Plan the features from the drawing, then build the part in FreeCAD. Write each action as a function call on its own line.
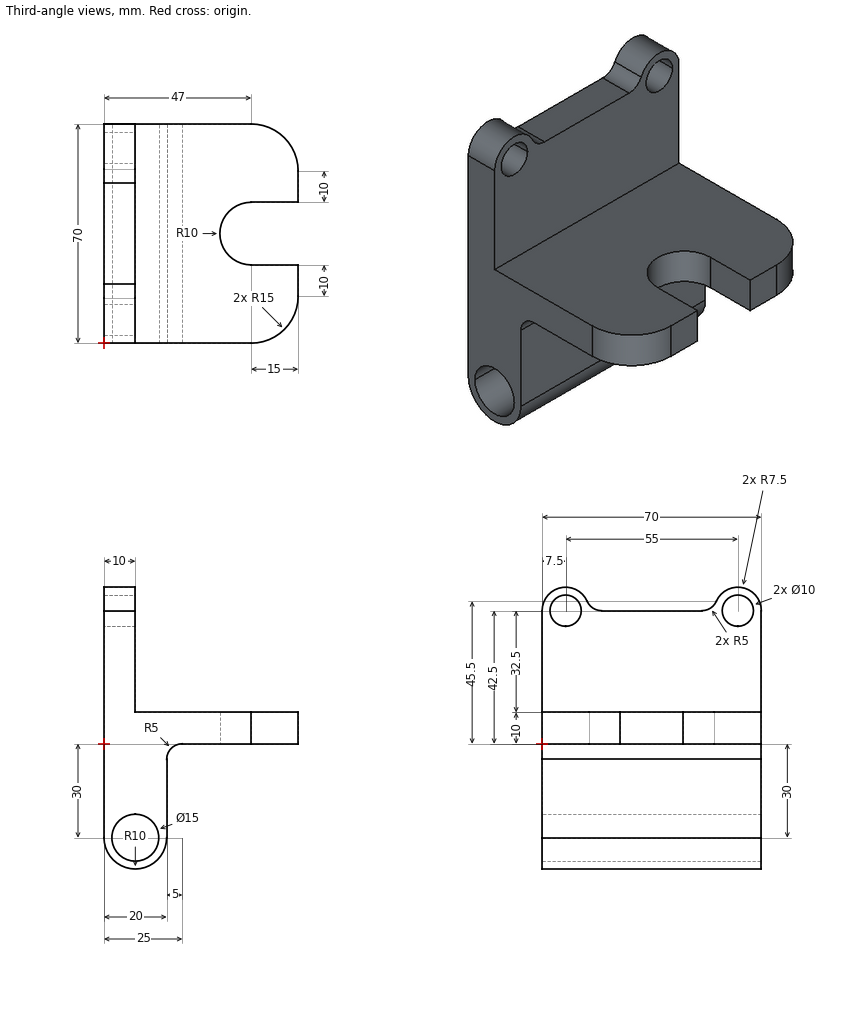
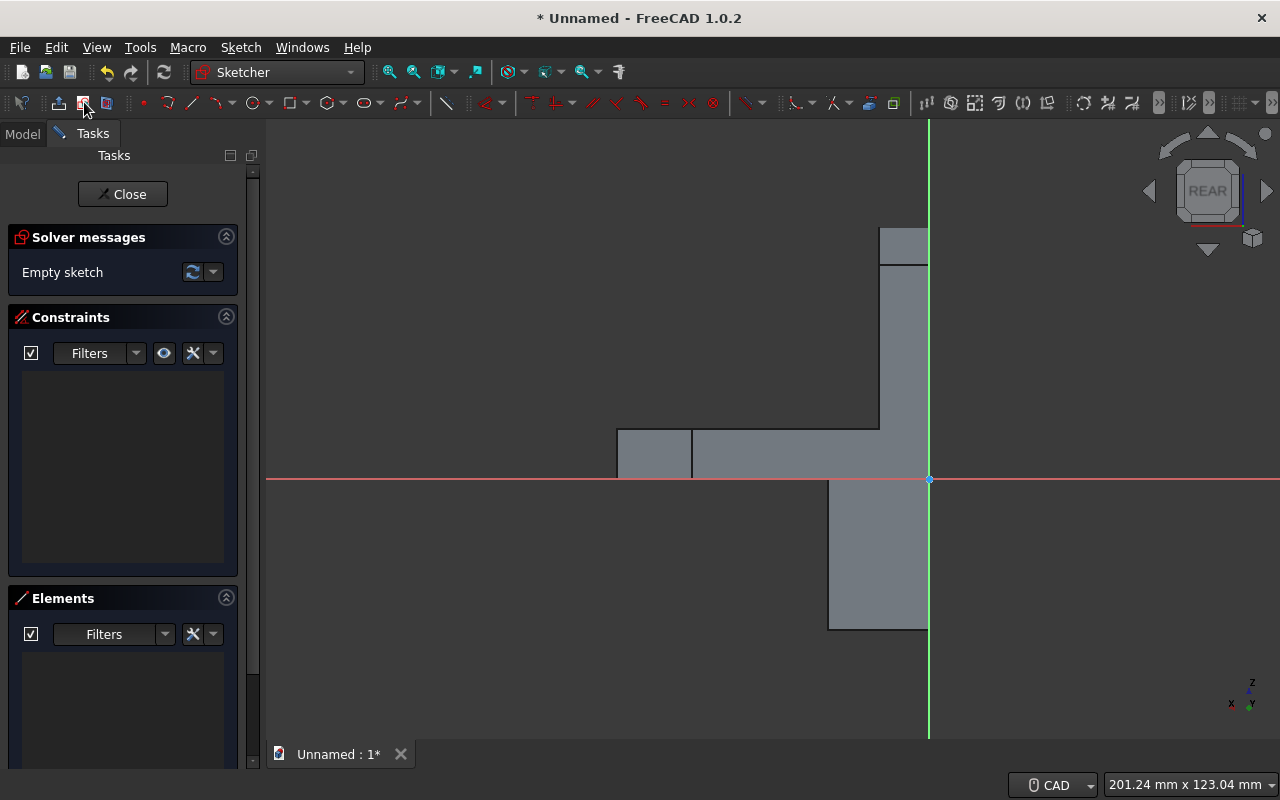
scroll(823, 496, up, 14)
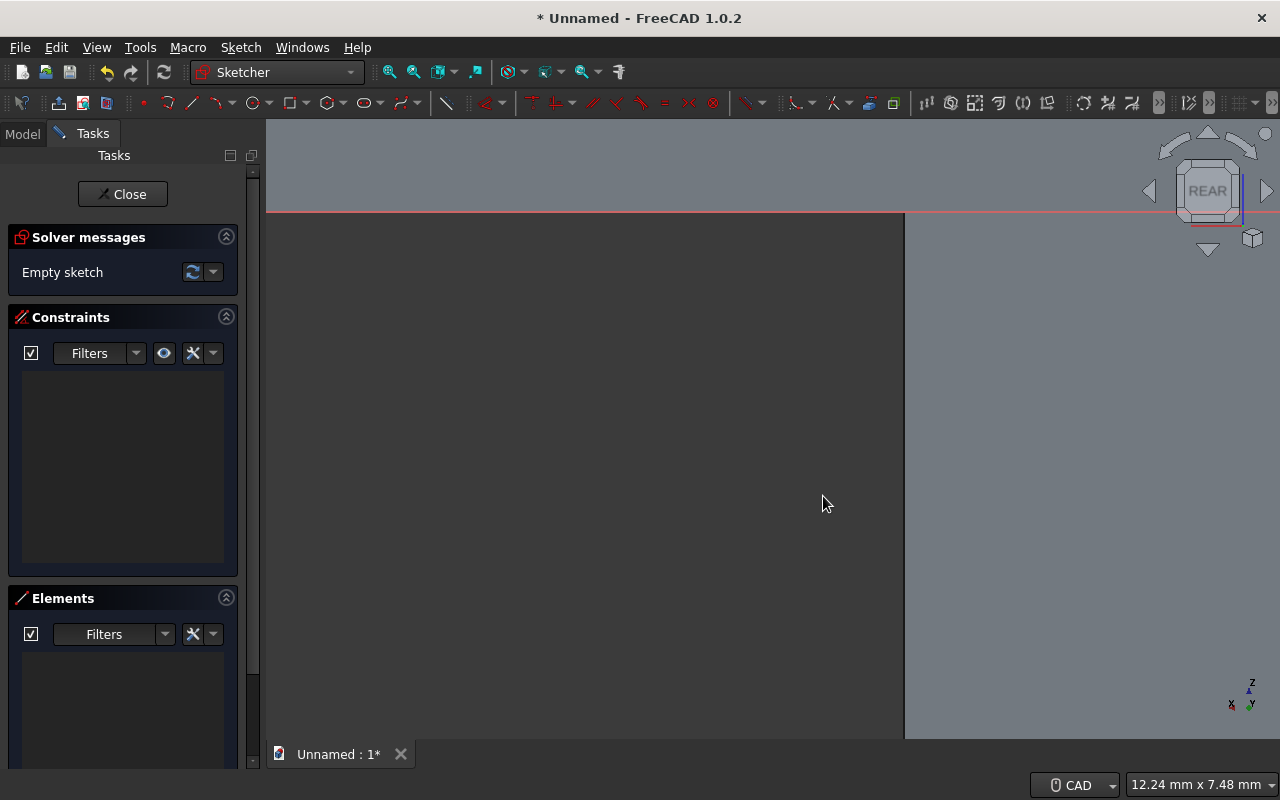
click(168, 104)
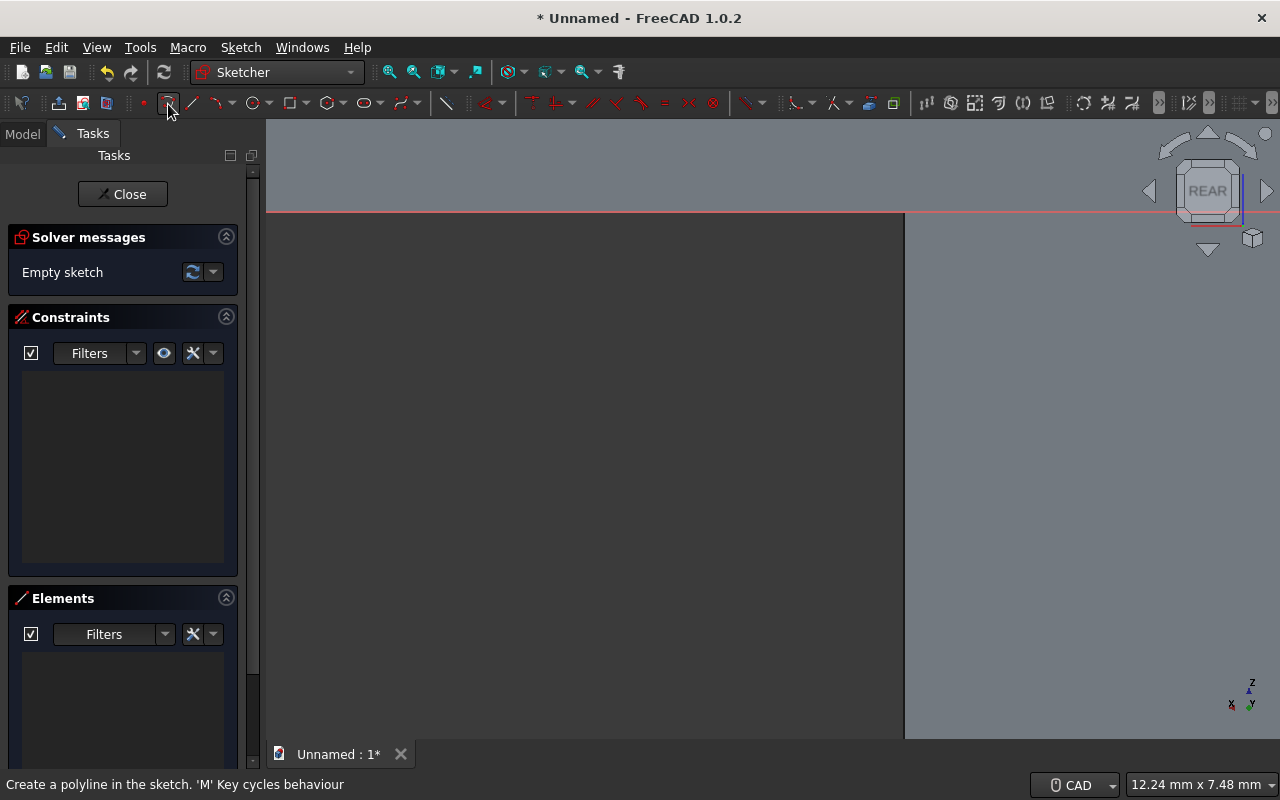
click(904, 627)
click(904, 212)
click(489, 221)
right_click(489, 221)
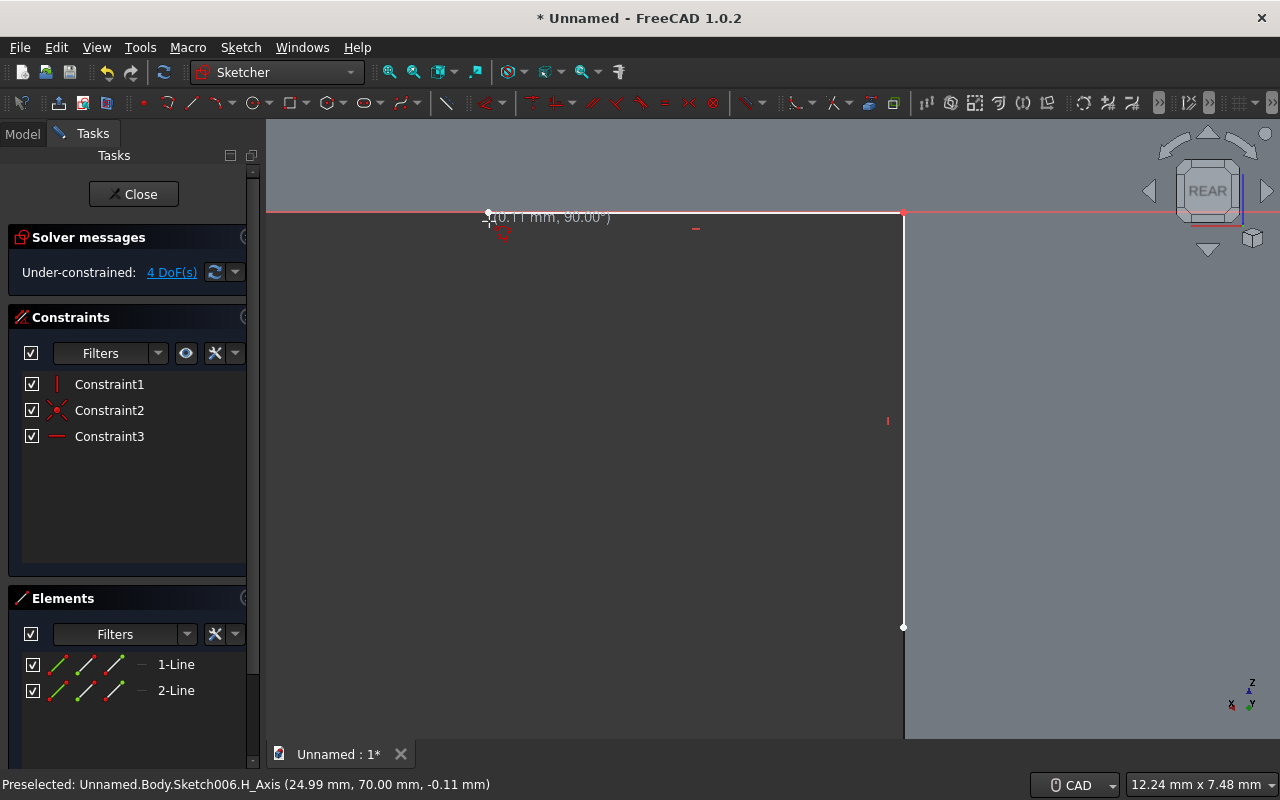
click(216, 104)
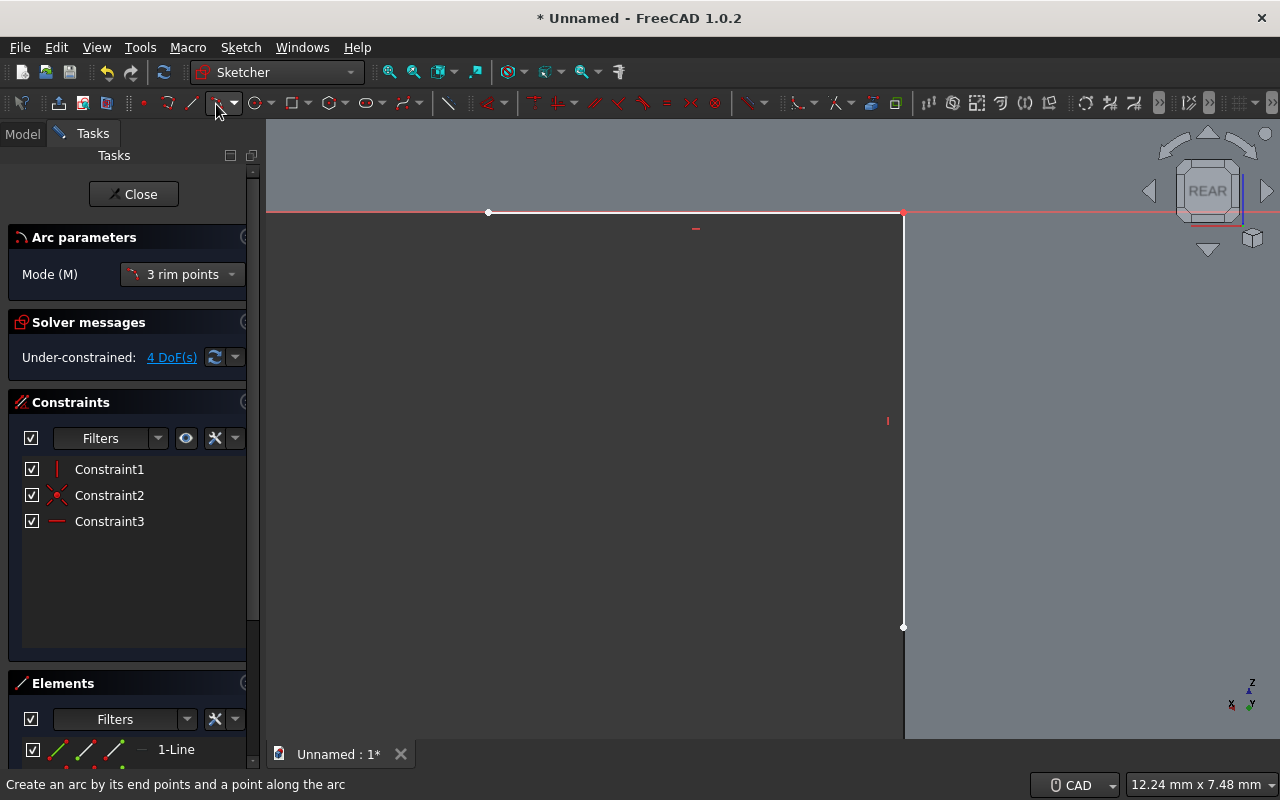
click(489, 213)
click(904, 628)
click(782, 334)
key(Escape)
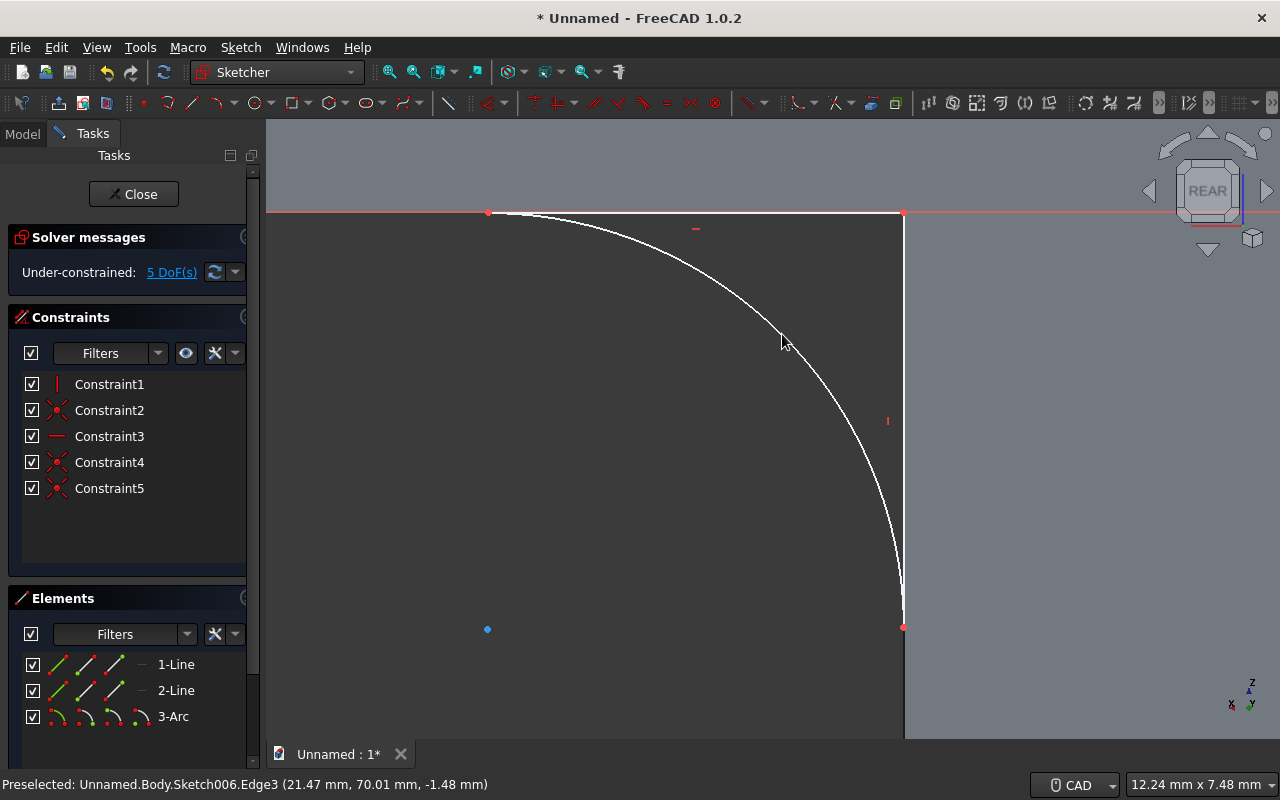
click(904, 503)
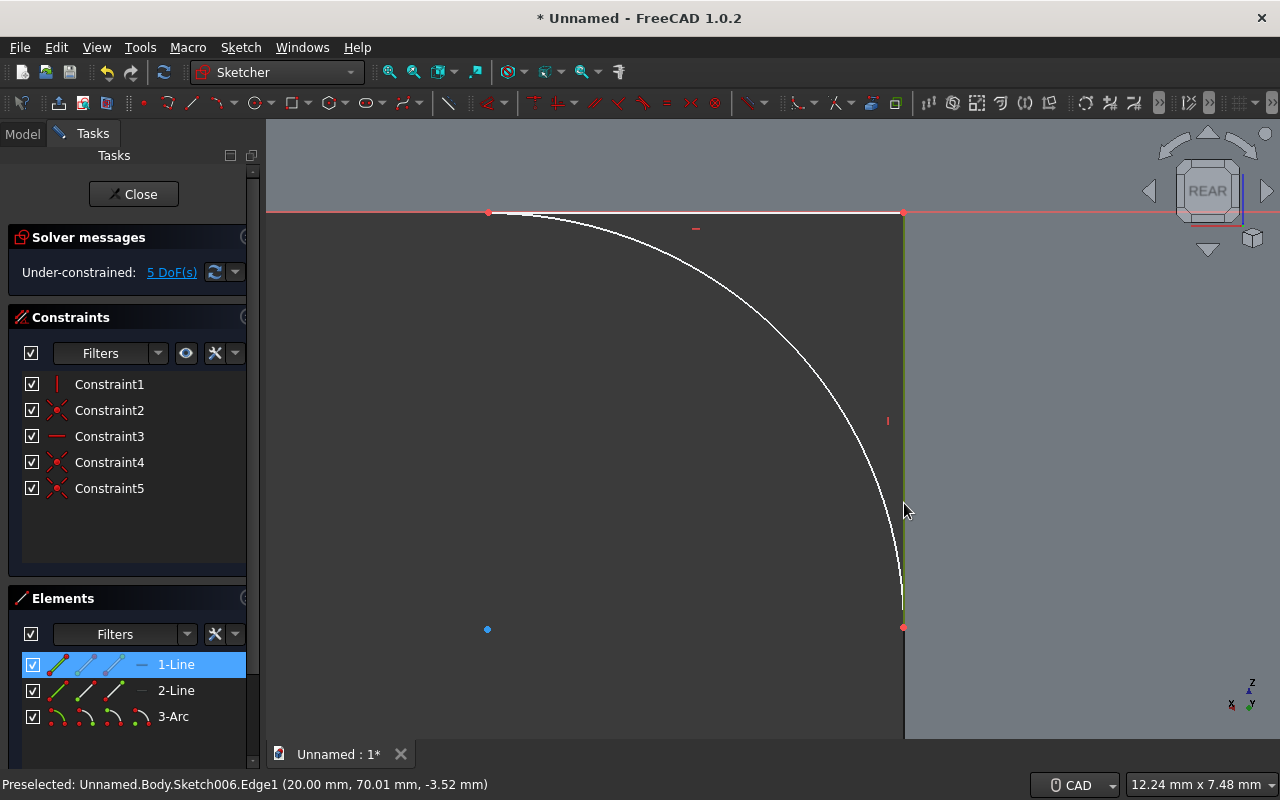
click(858, 440)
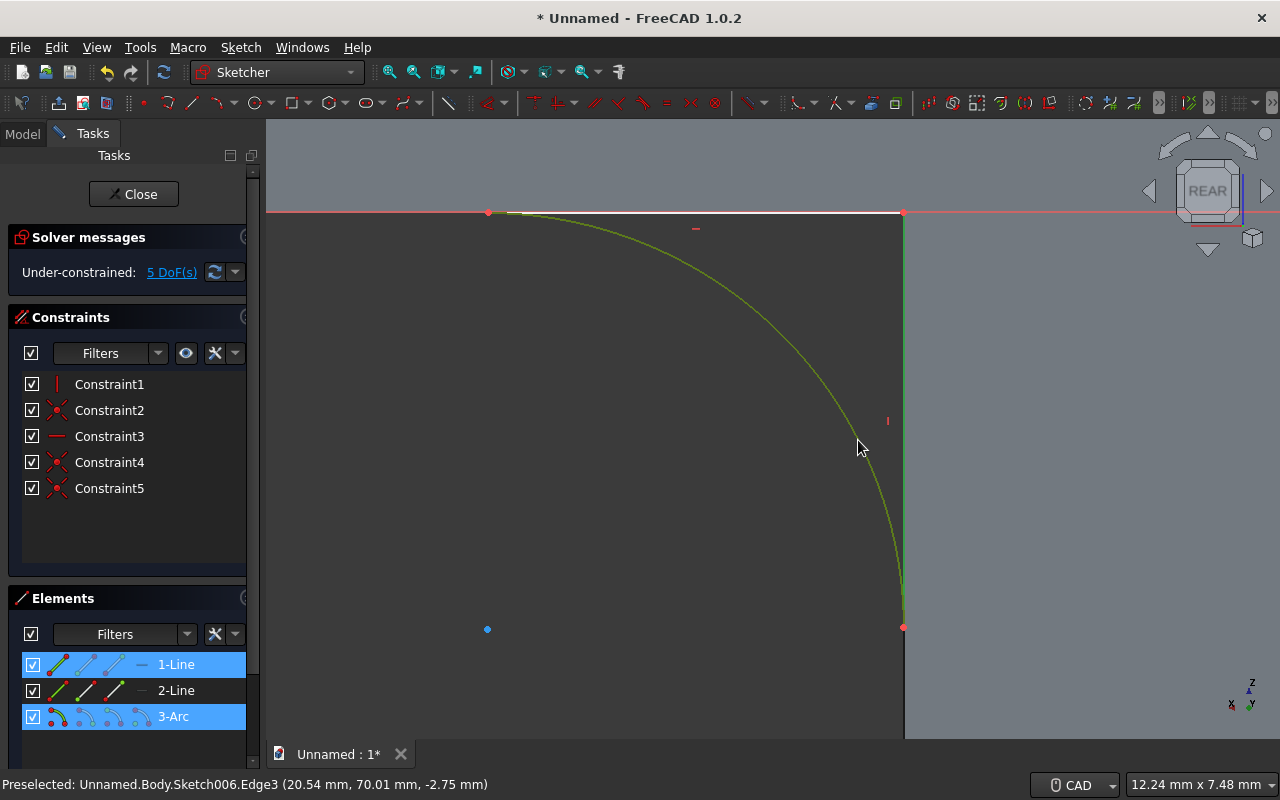
click(644, 104)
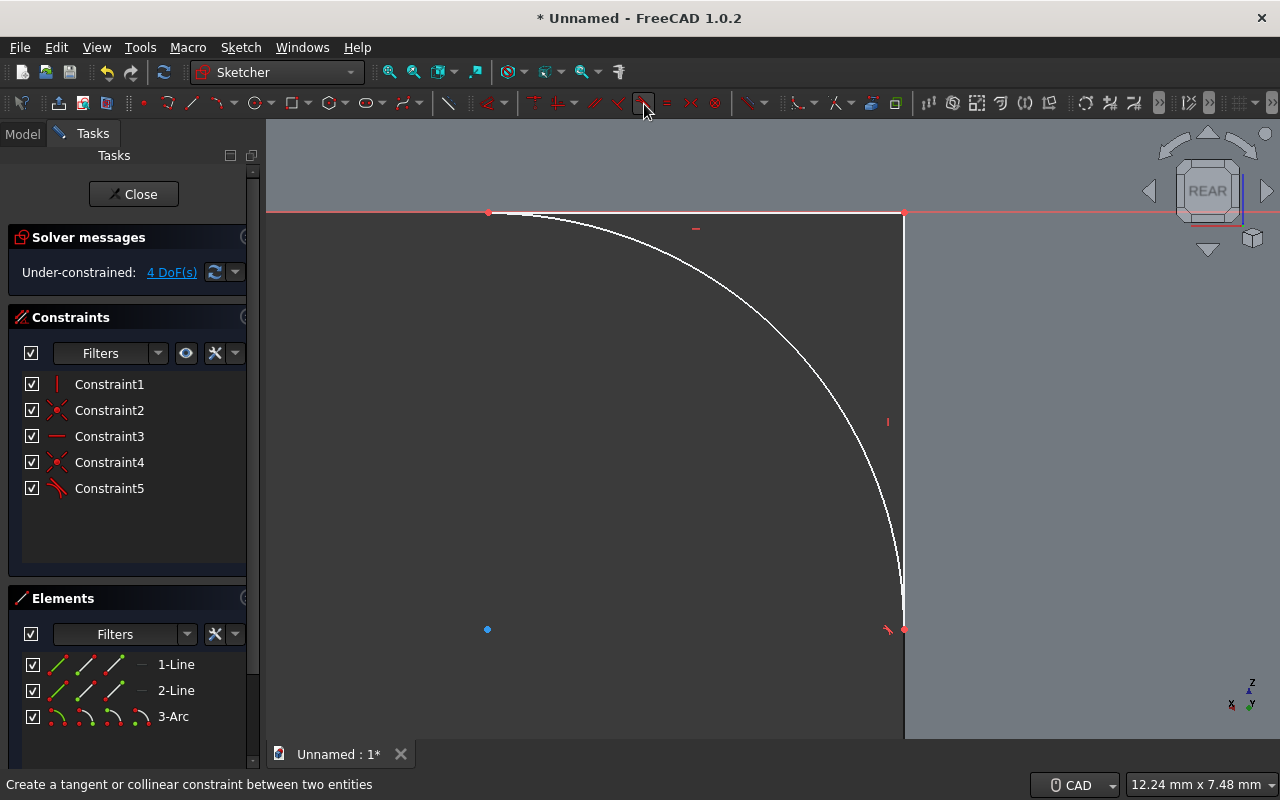
click(780, 213)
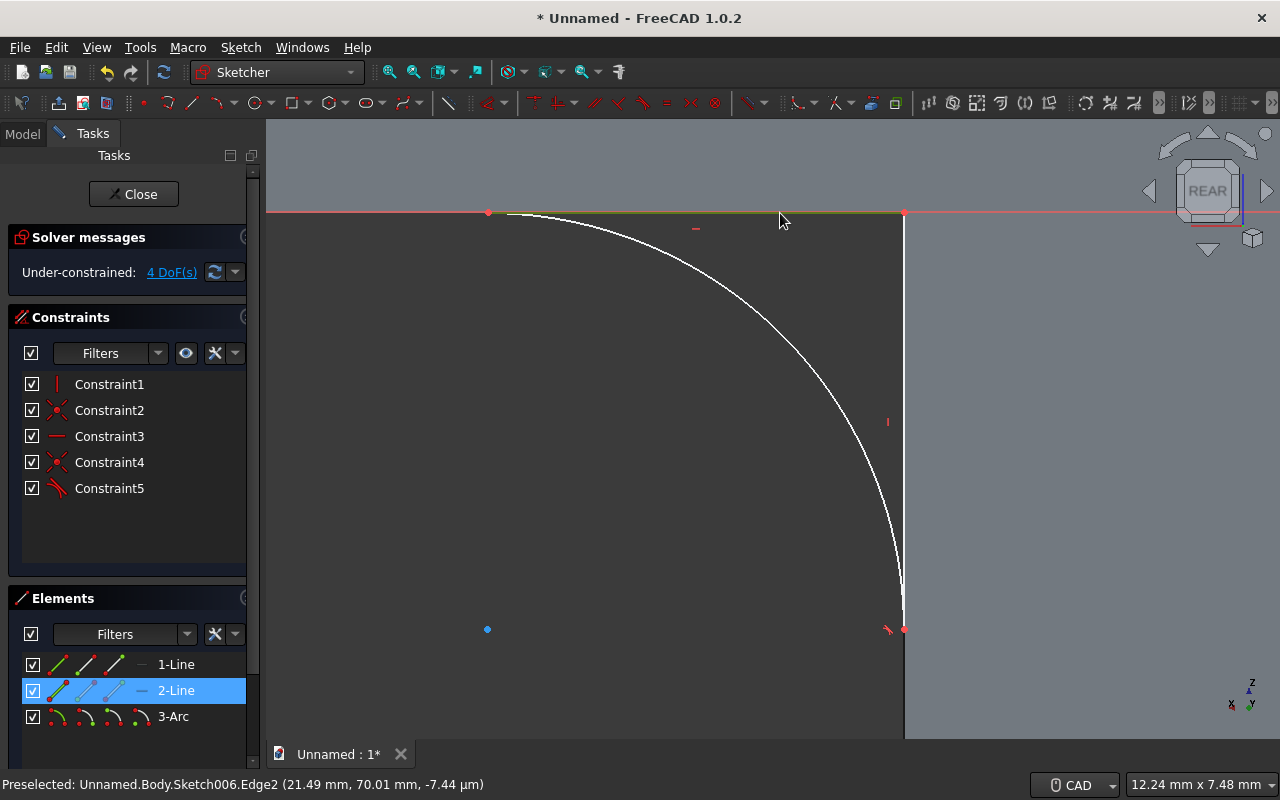
click(859, 441)